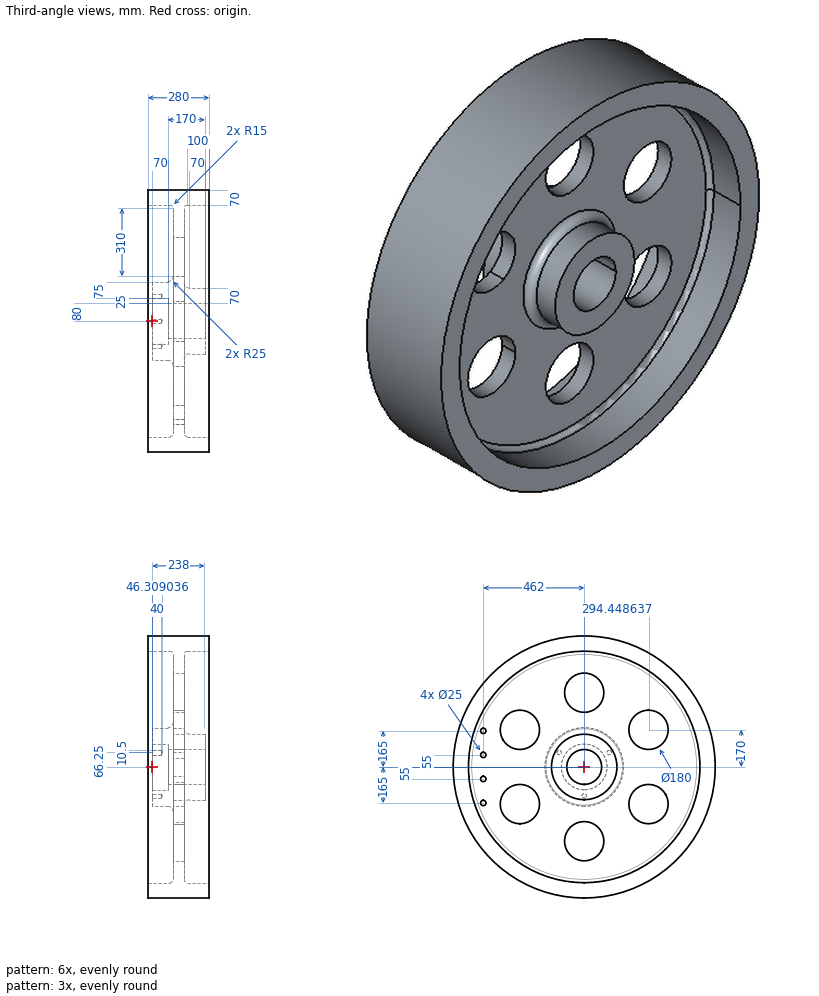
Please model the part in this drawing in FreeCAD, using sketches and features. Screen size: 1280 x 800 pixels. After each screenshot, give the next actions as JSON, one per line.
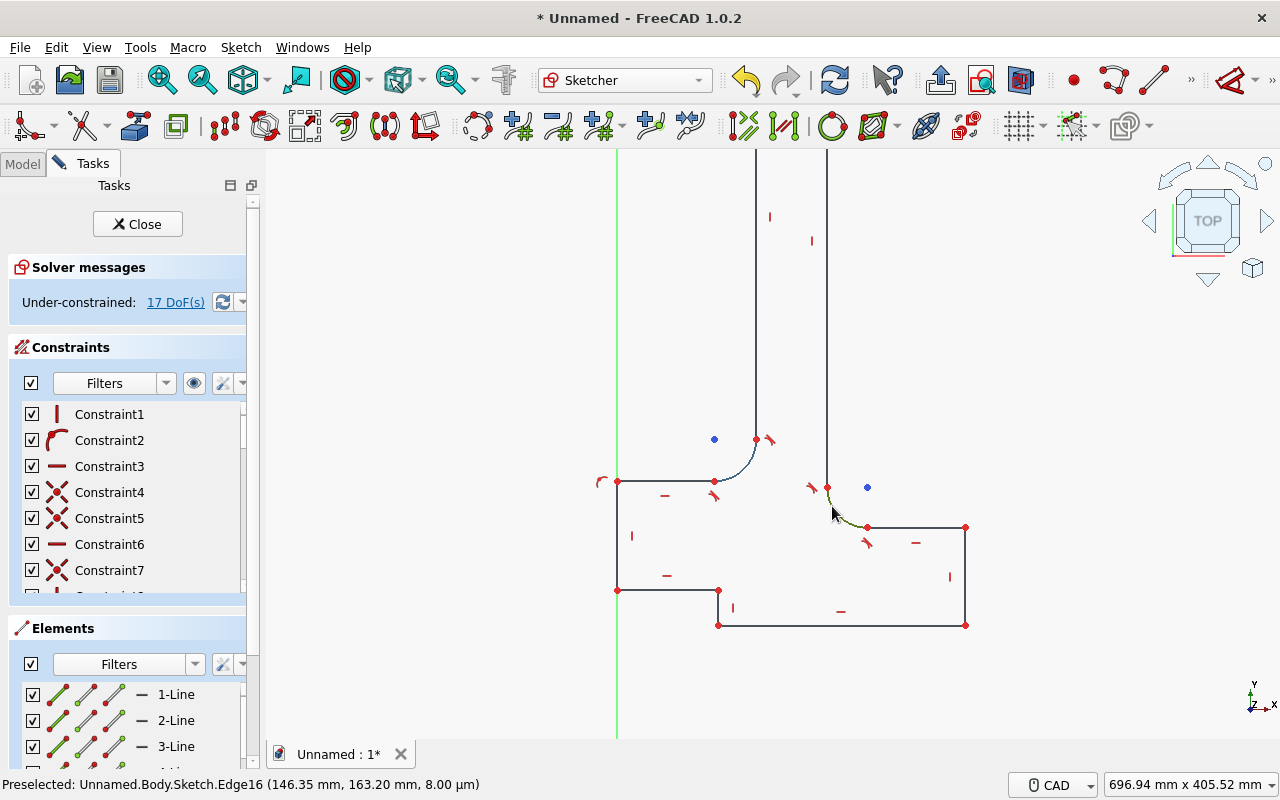
{"action": "key", "text": "e"}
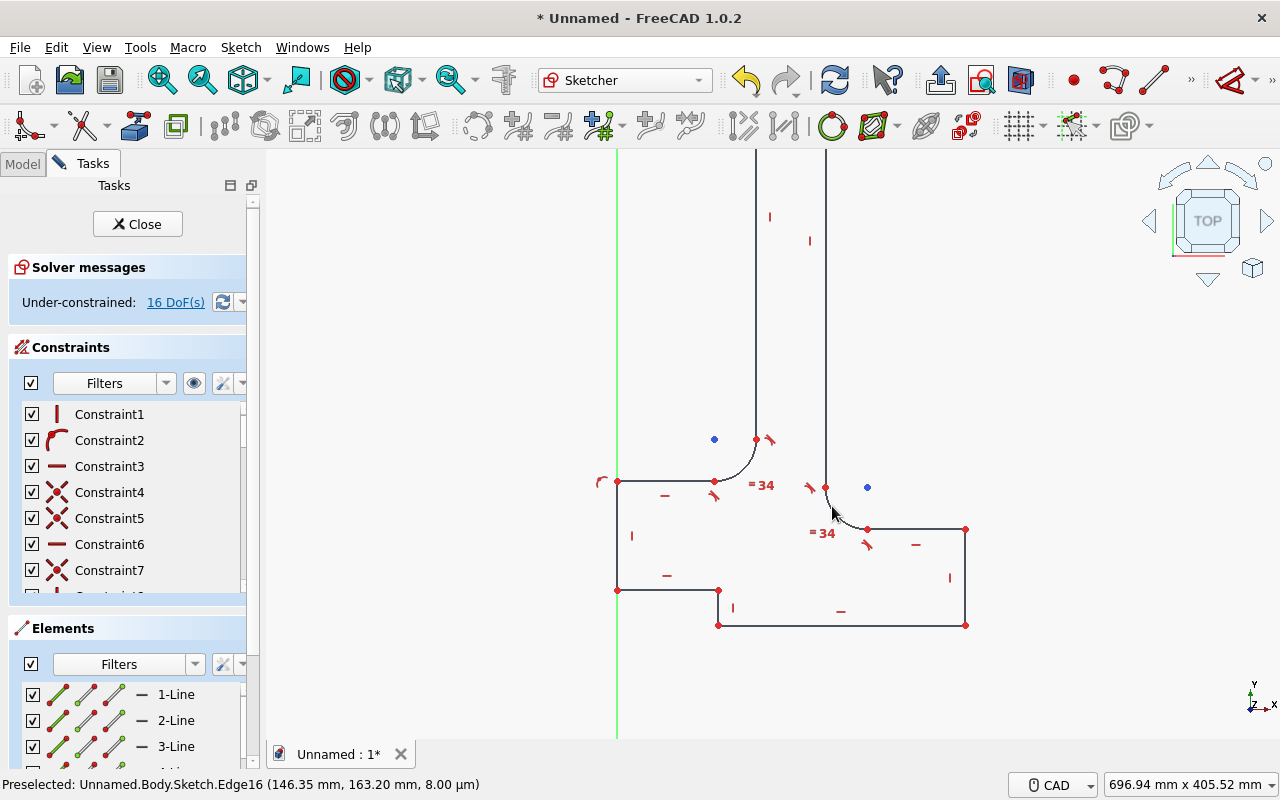
{"action": "scroll", "coordinate": [633, 559], "scroll_direction": "down", "scroll_amount": 4}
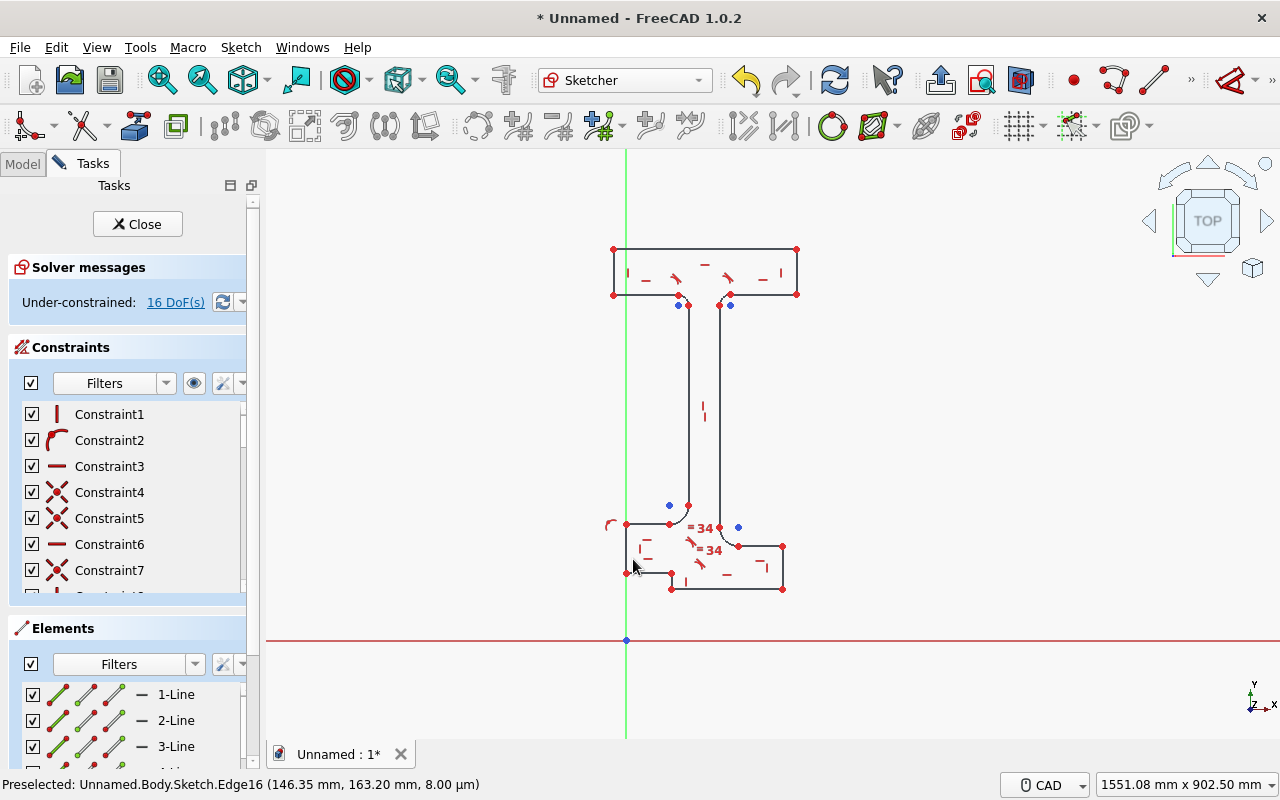
{"action": "scroll", "coordinate": [726, 296], "scroll_direction": "up", "scroll_amount": 6}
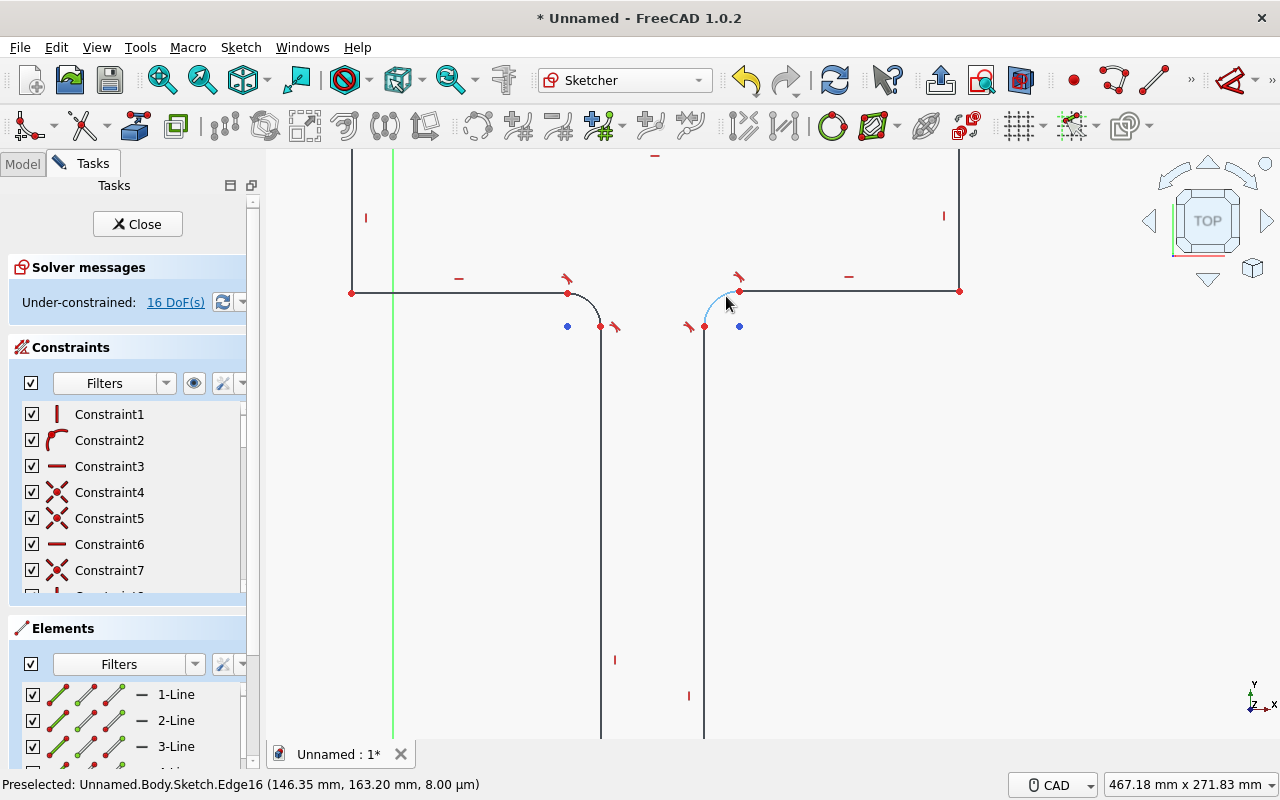
{"action": "left_click", "coordinate": [724, 295]}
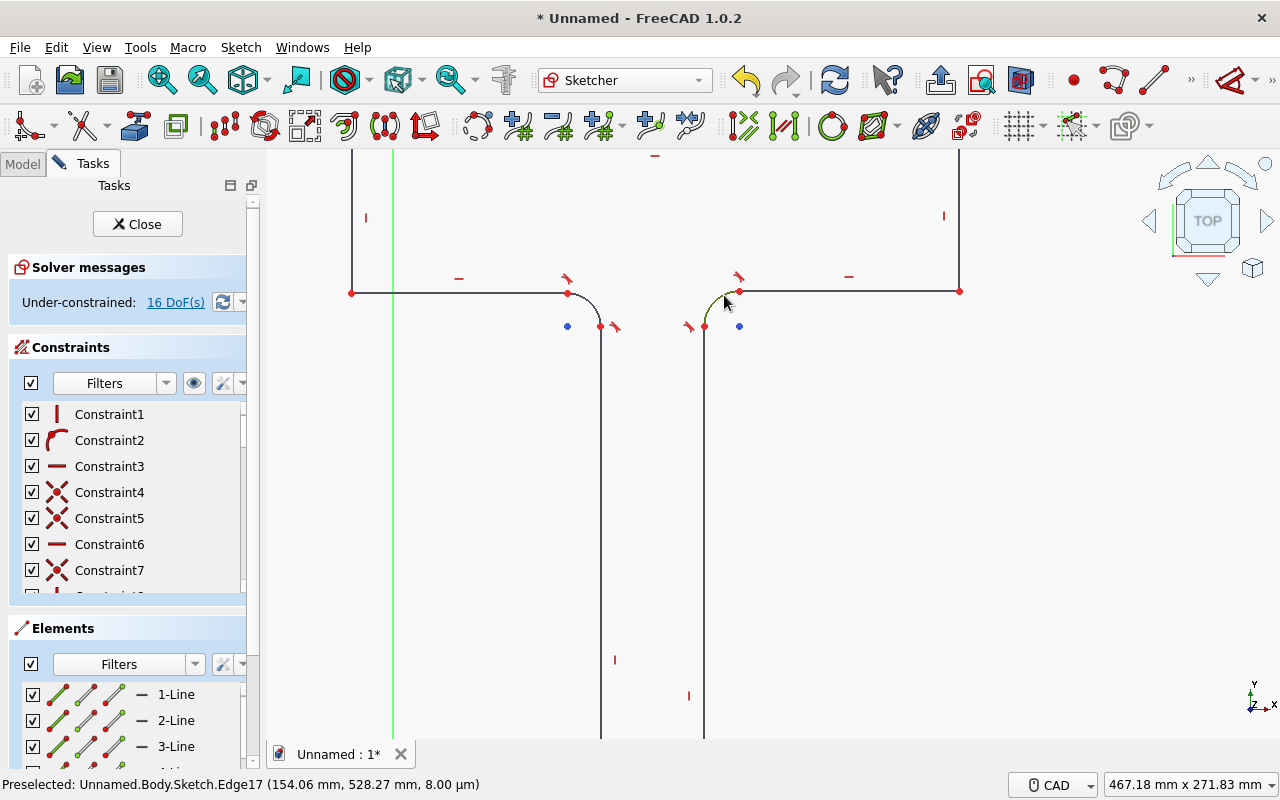
{"action": "left_click", "coordinate": [597, 312]}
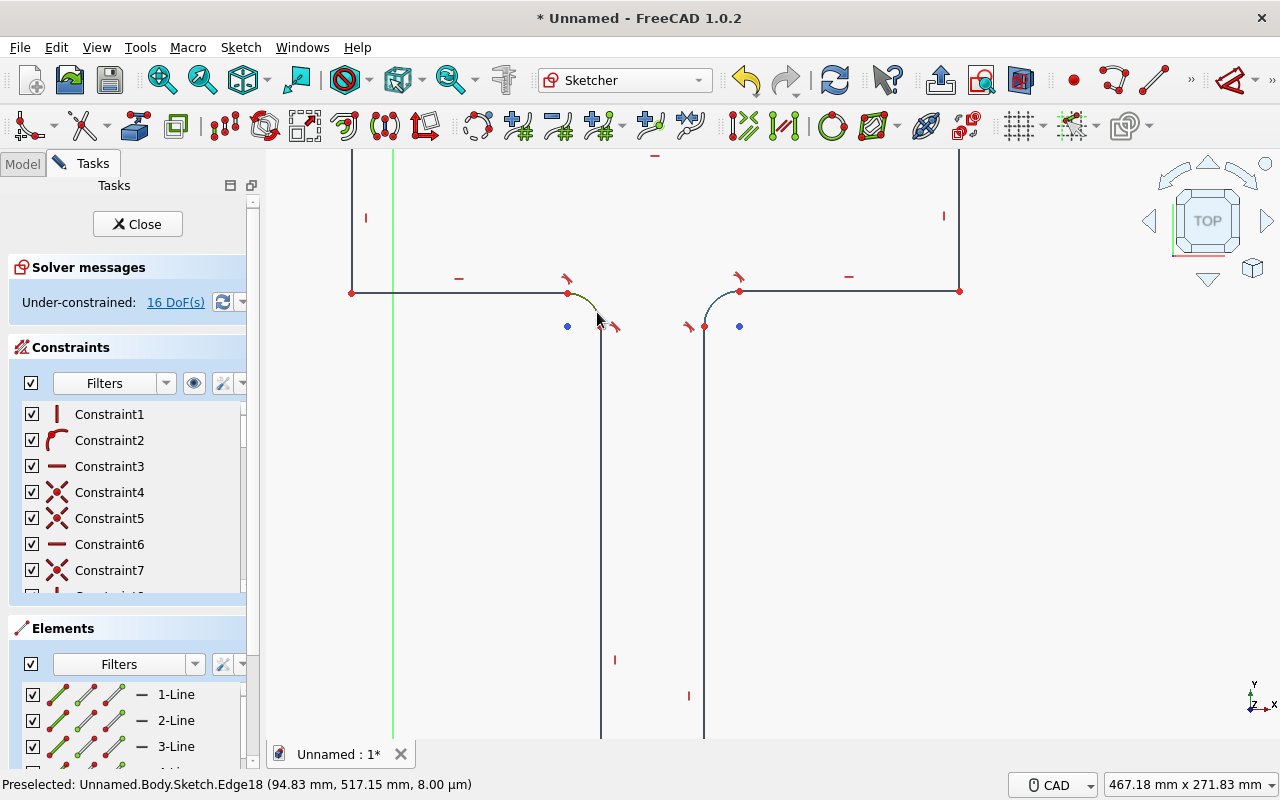
{"action": "key", "text": "e"}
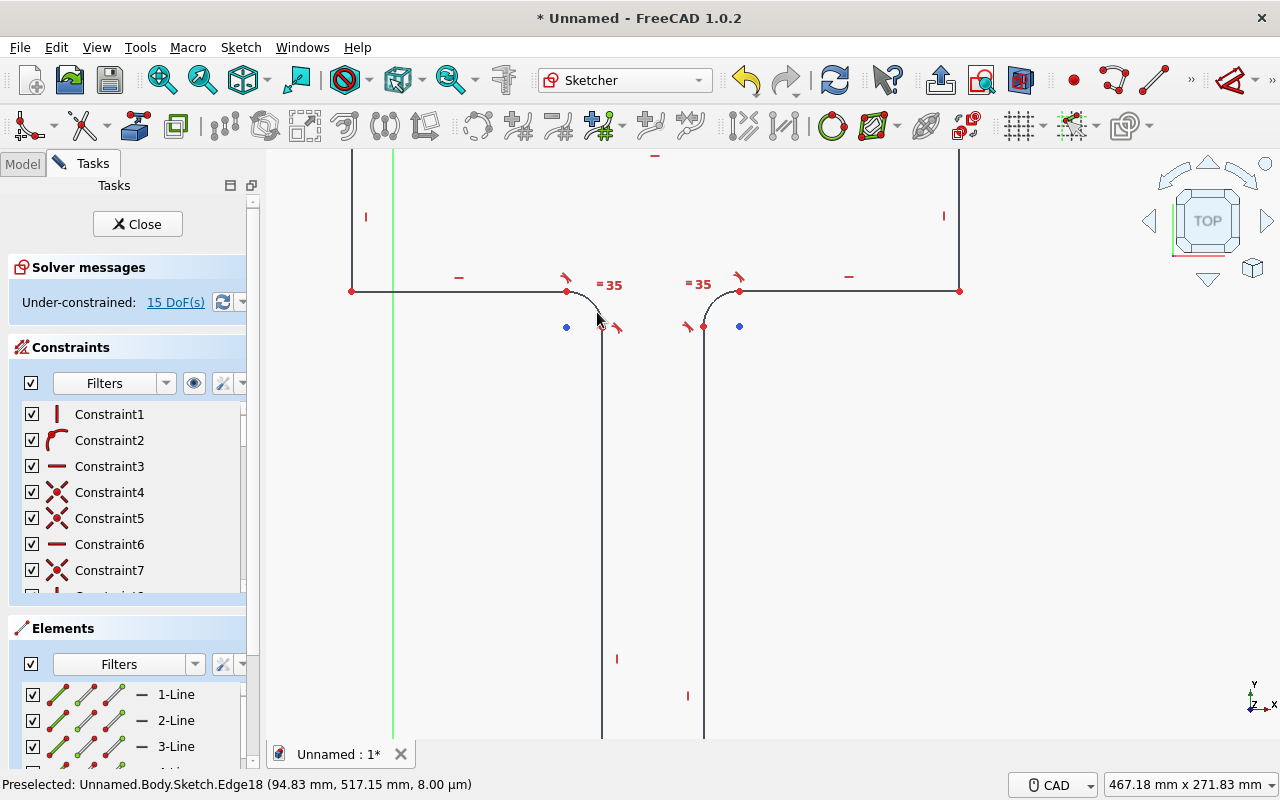
{"action": "scroll", "coordinate": [726, 295], "scroll_direction": "down", "scroll_amount": 6}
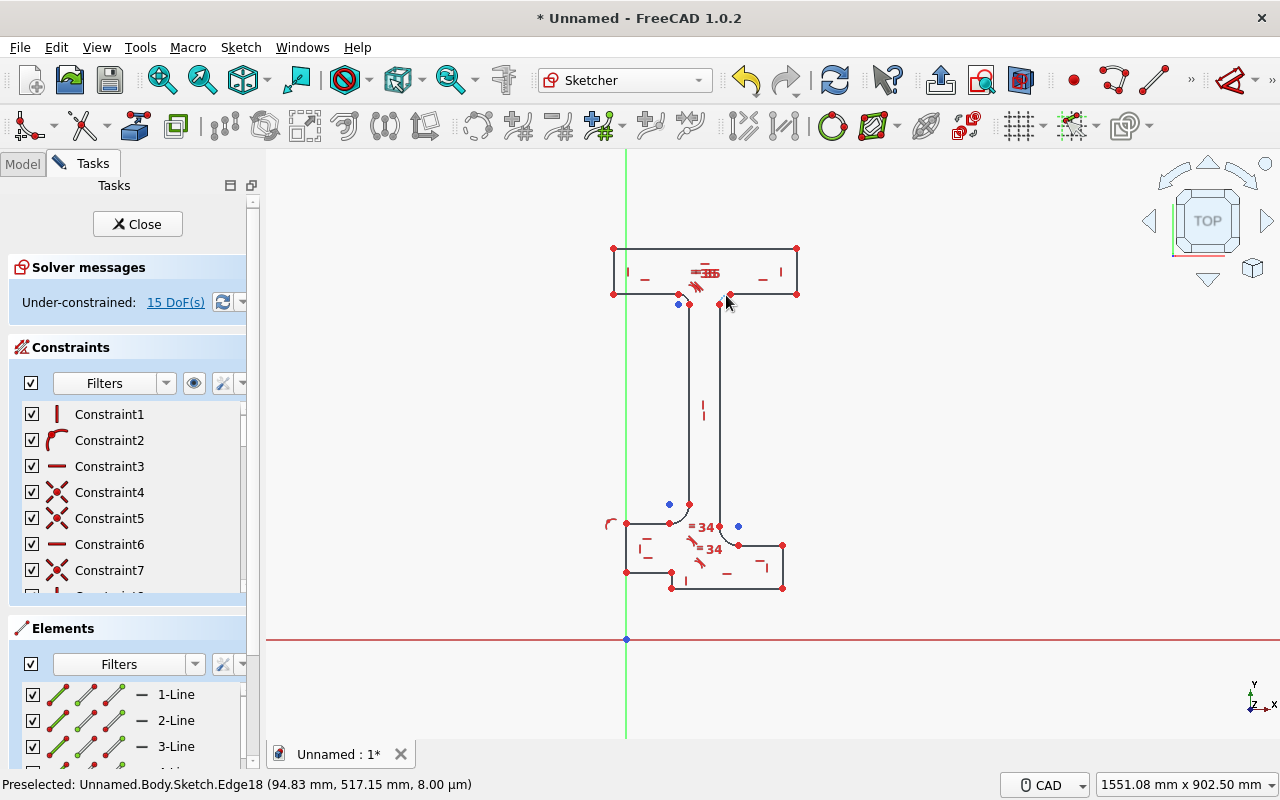
{"action": "scroll", "coordinate": [679, 522], "scroll_direction": "up", "scroll_amount": 5}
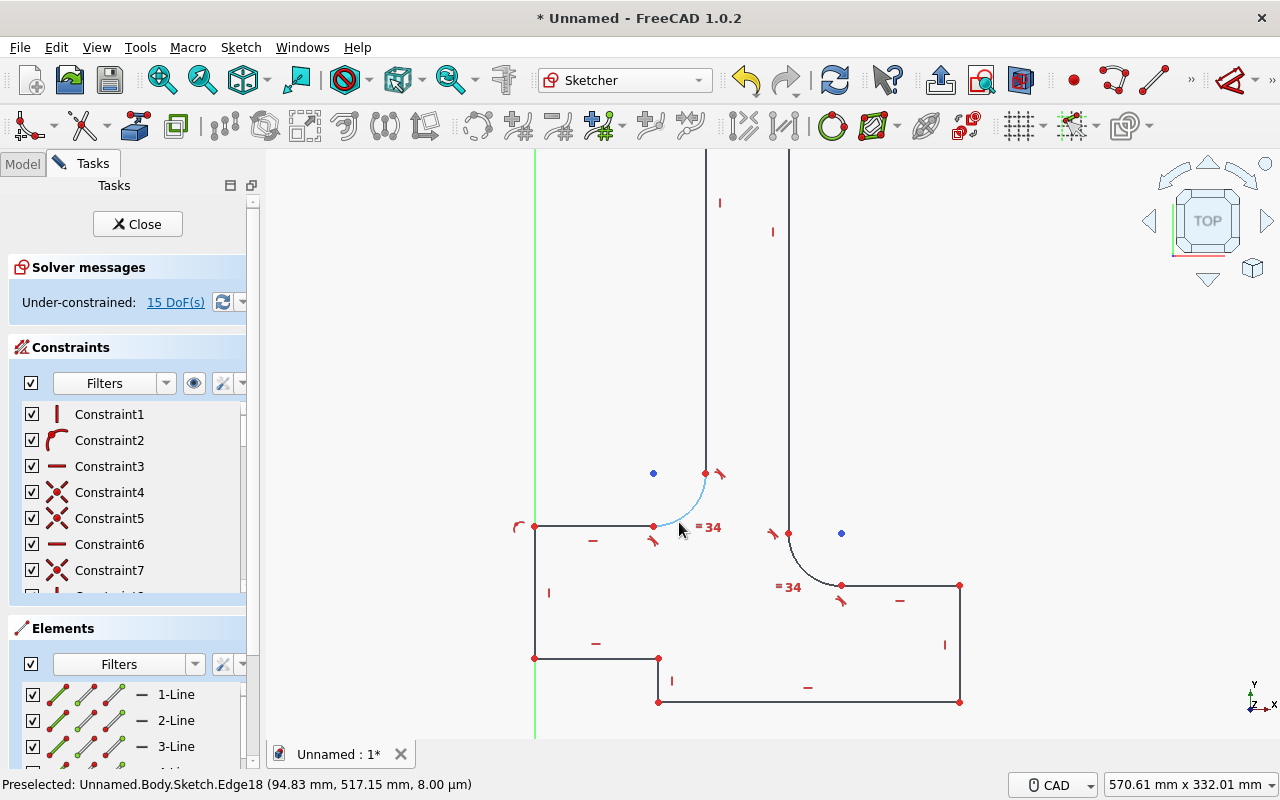
{"action": "left_click", "coordinate": [677, 520]}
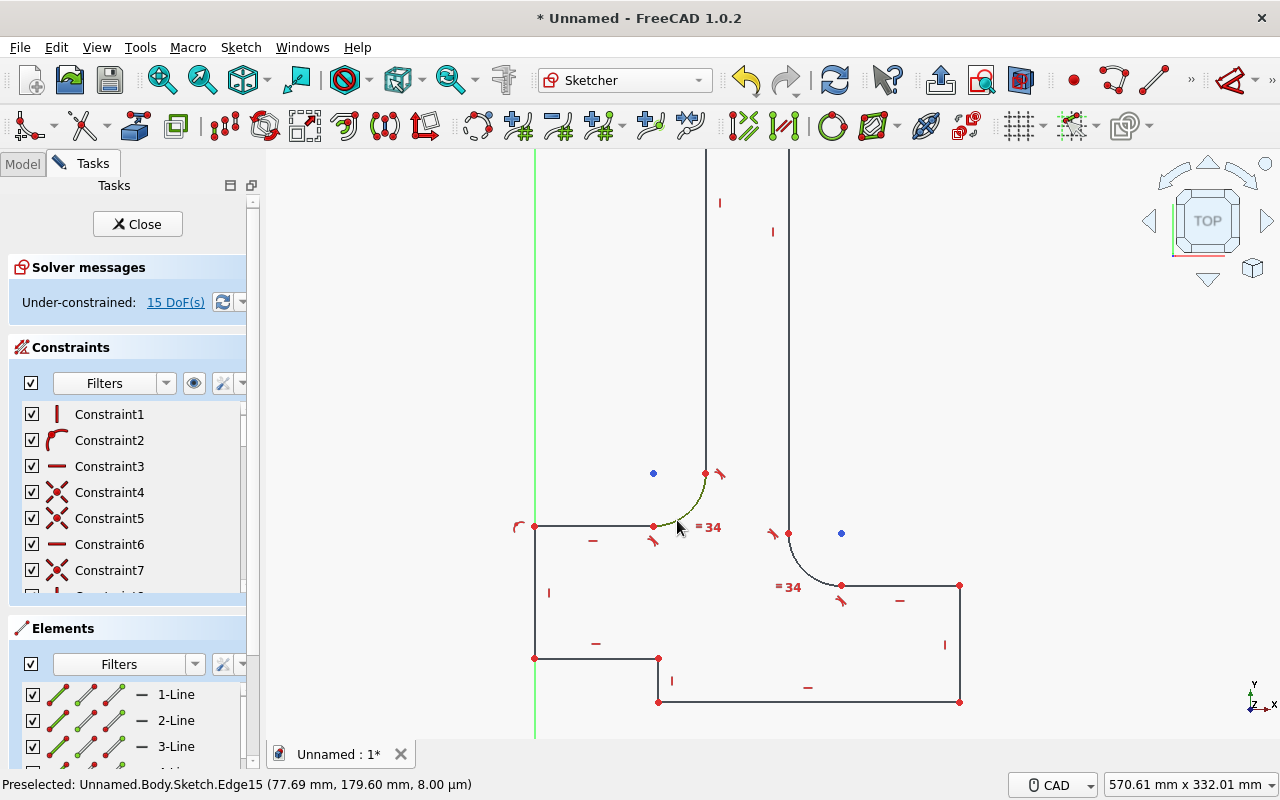
{"action": "key", "text": "k r"}